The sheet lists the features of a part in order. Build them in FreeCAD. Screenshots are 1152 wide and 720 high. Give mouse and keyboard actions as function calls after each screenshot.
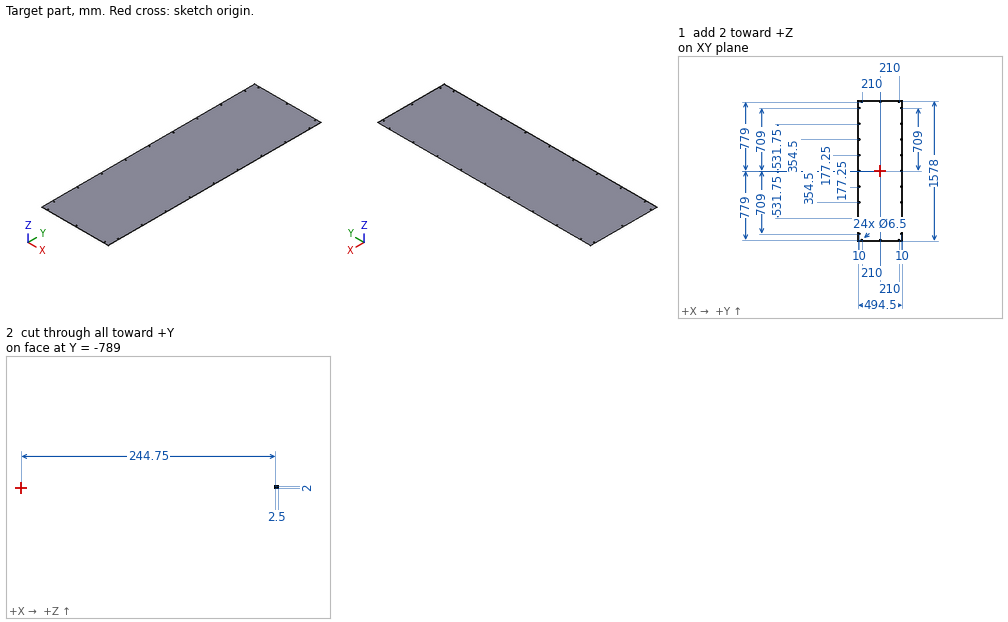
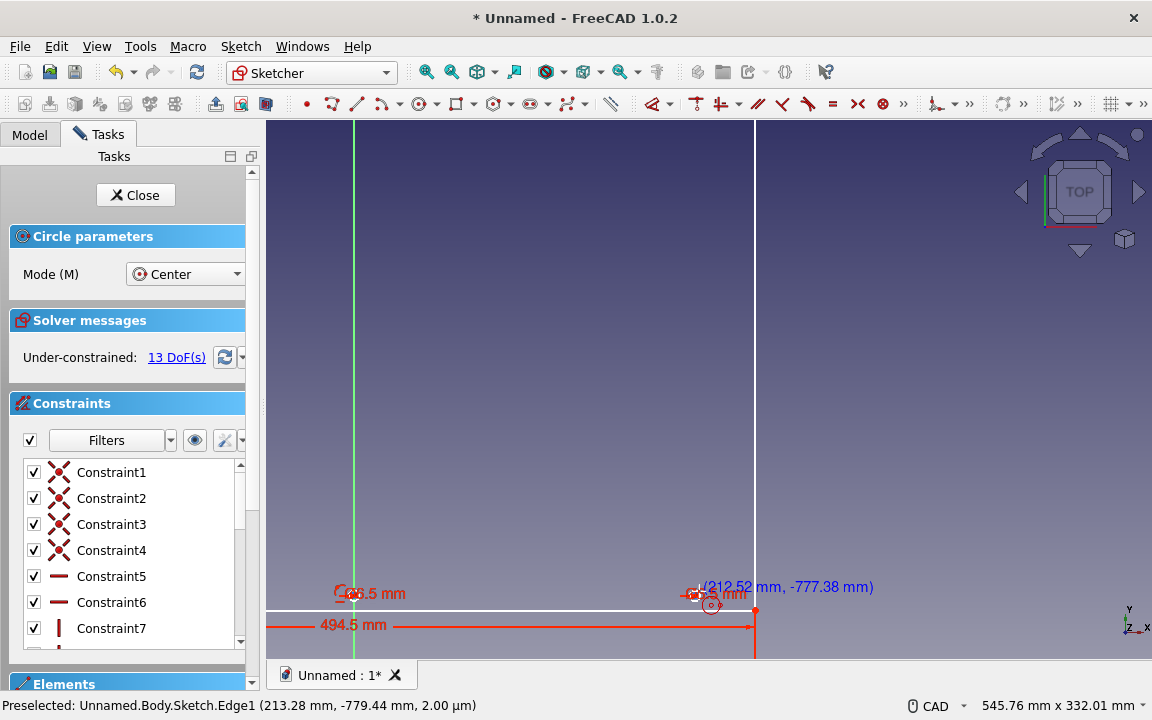
scroll(739, 481, up, 8)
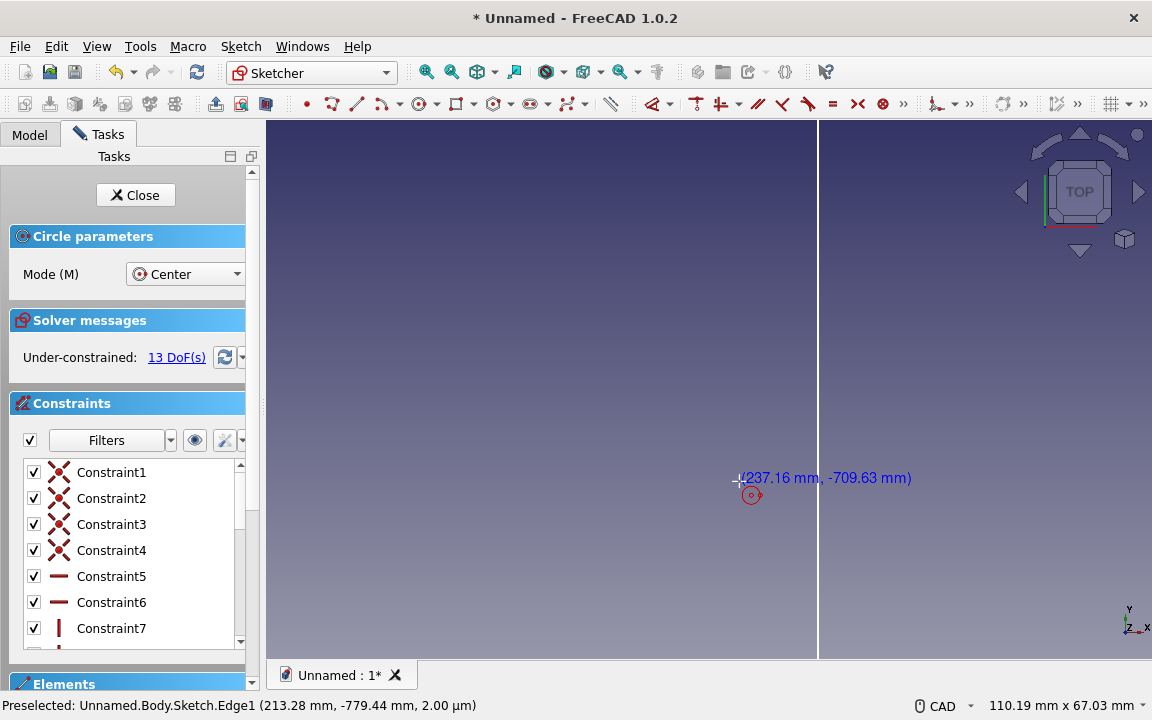
scroll(703, 583, down, 17)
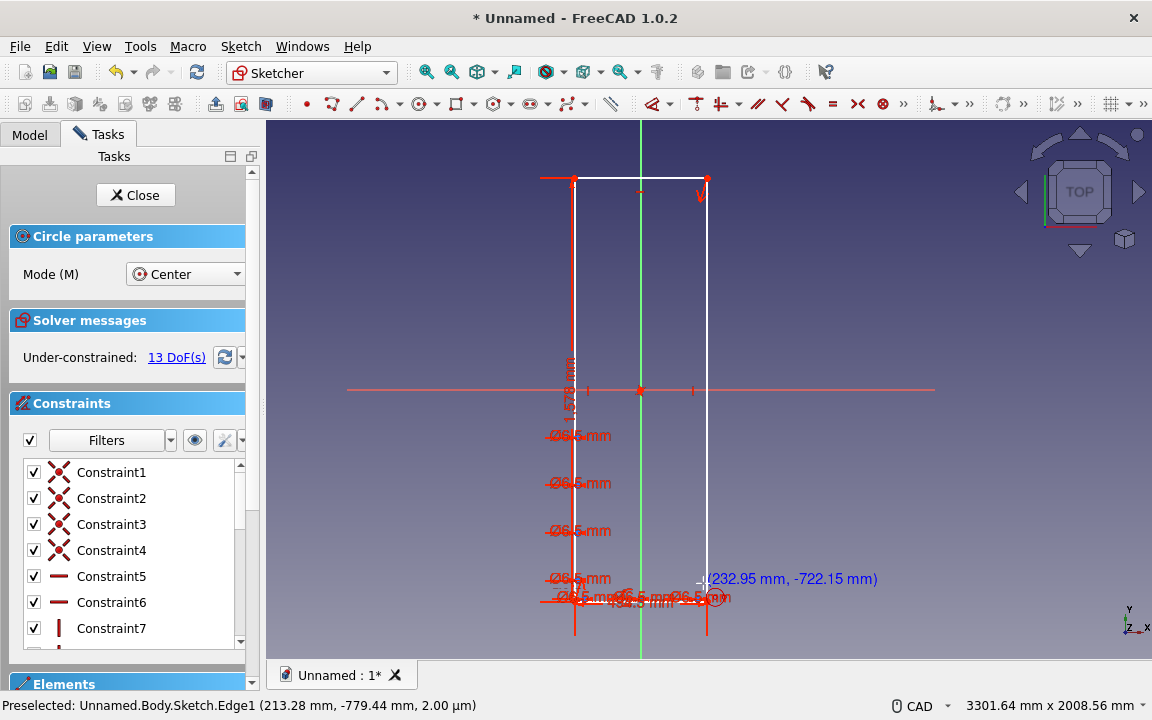
scroll(705, 580, up, 9)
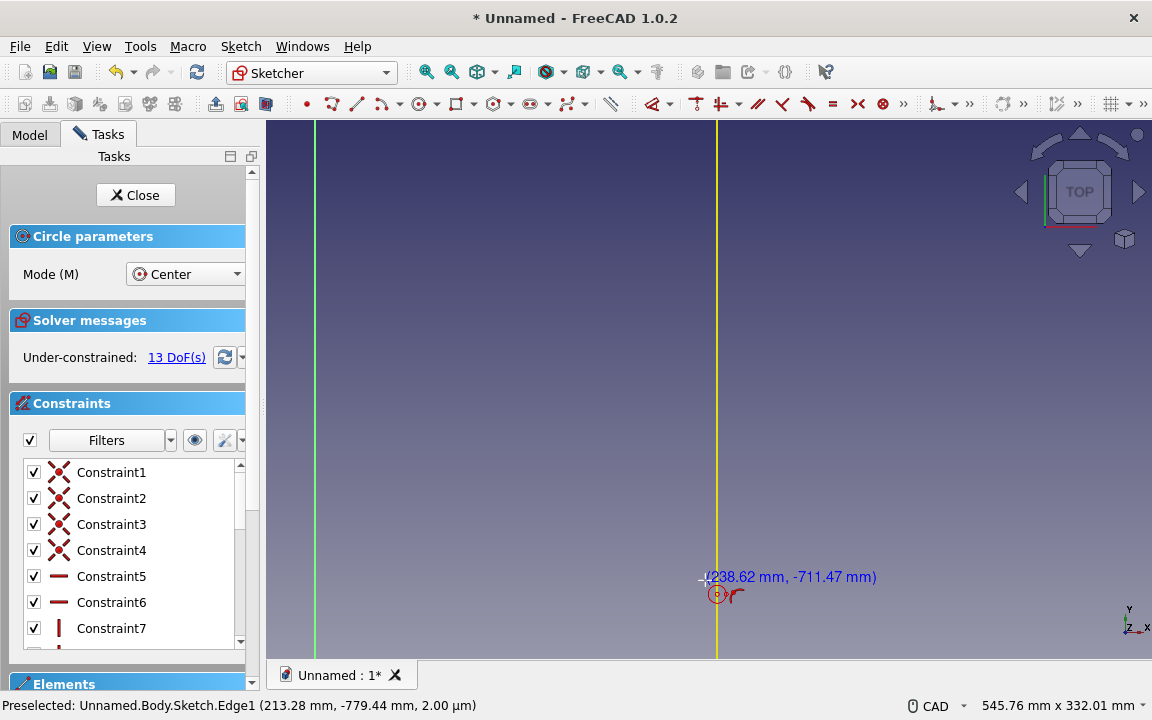
click(700, 578)
move(697, 574)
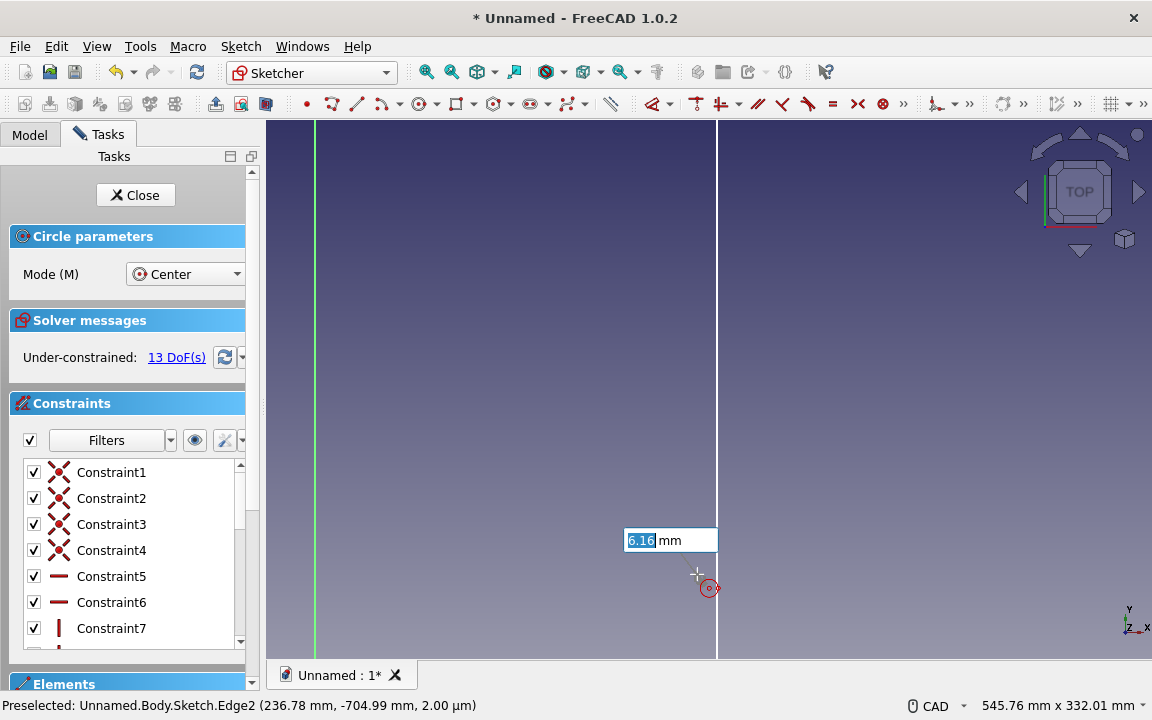
text(6.5)
key(Return)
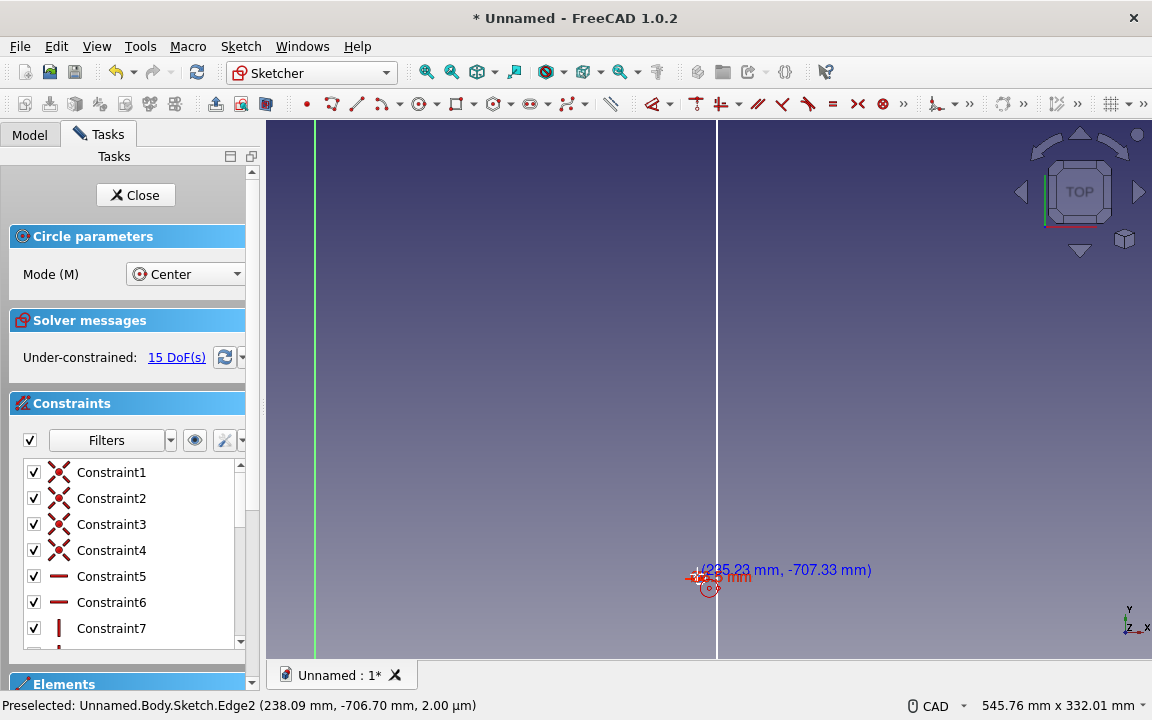
scroll(700, 290, up, 8)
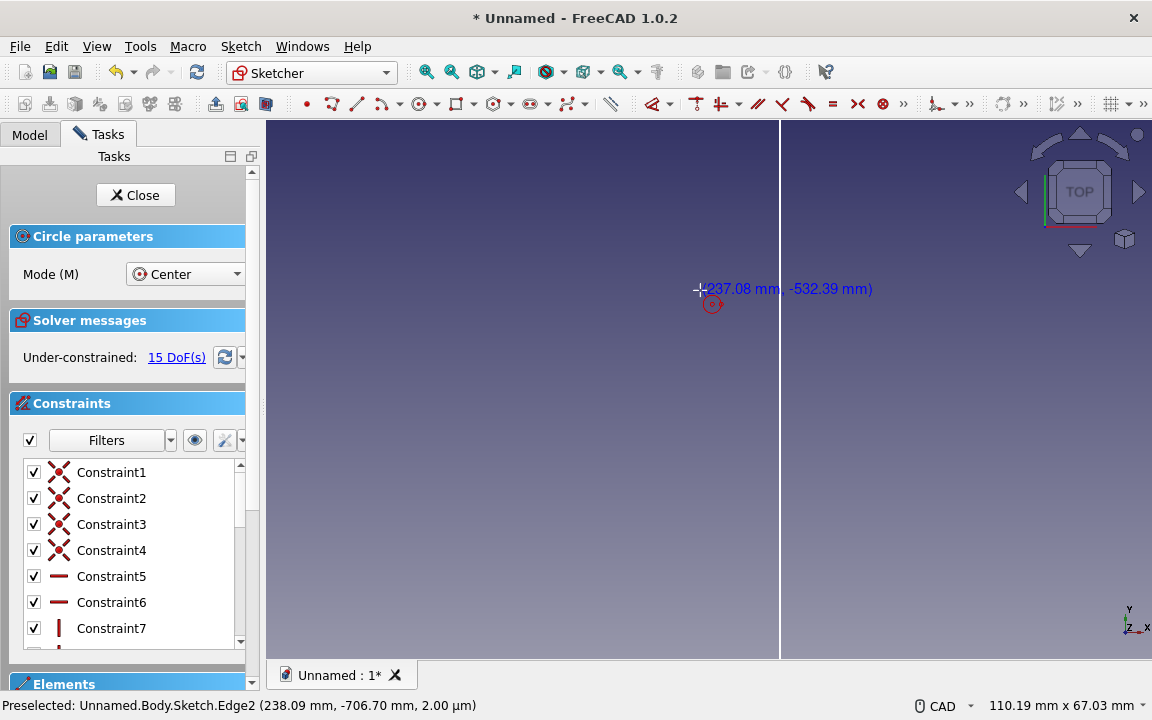
scroll(704, 541, down, 17)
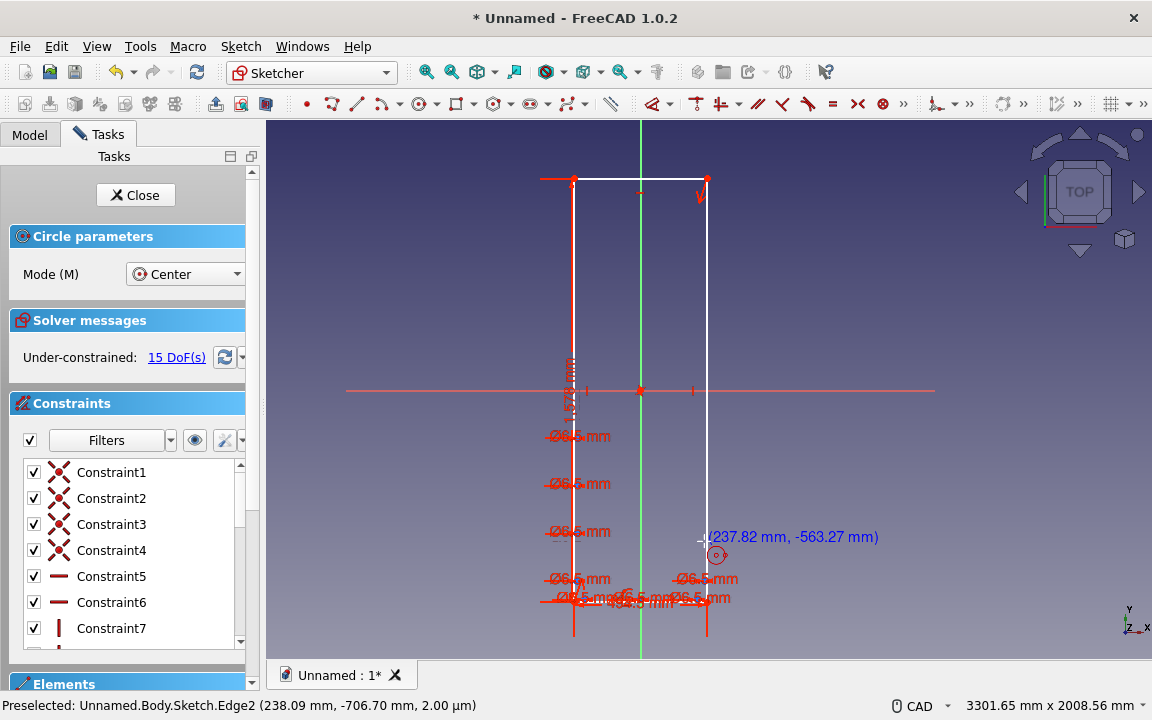
scroll(704, 533, up, 9)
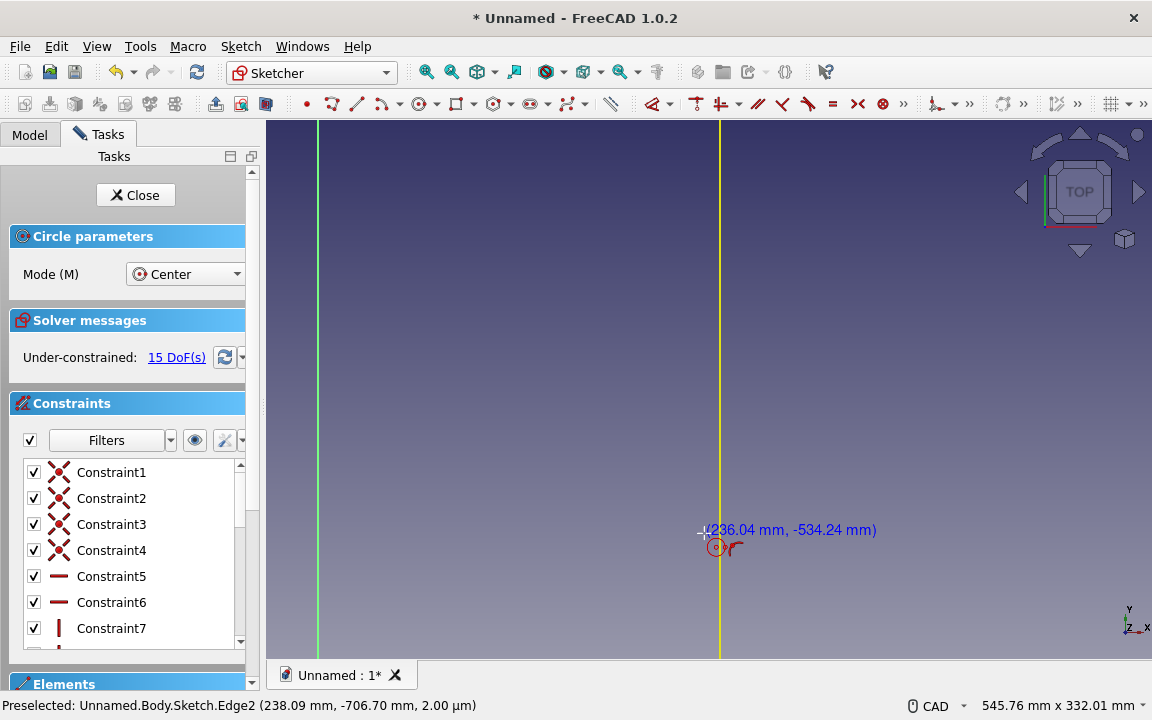
click(703, 531)
move(700, 527)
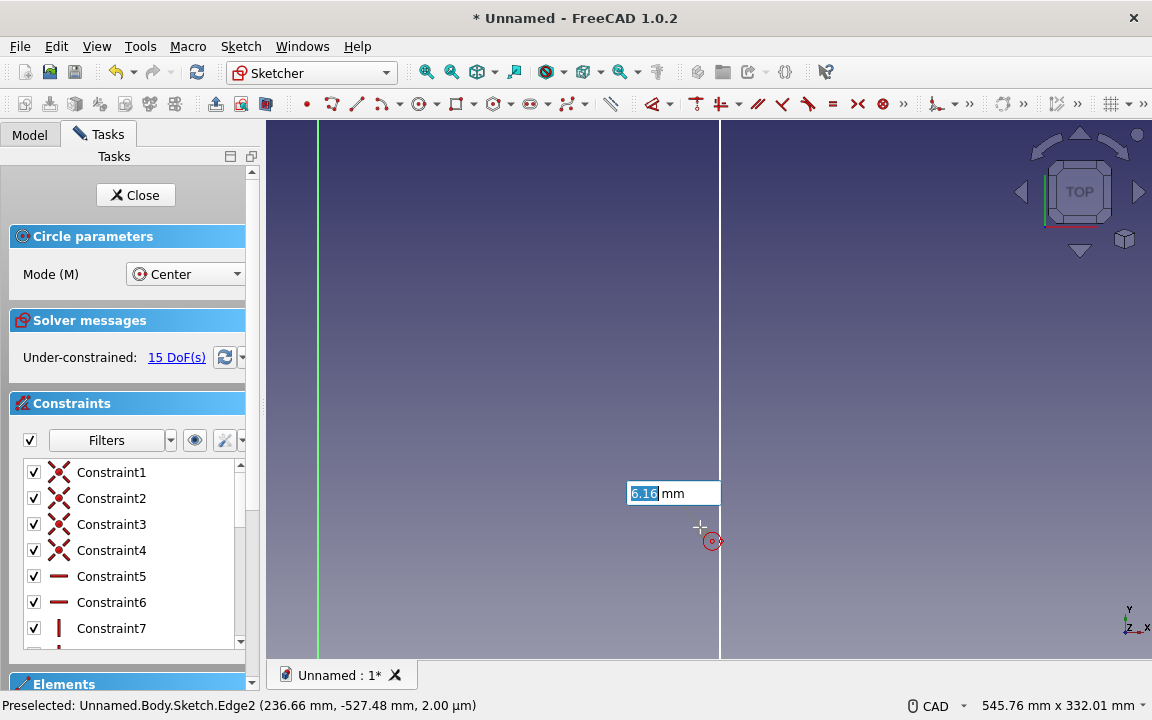
text(6.5)
key(Return)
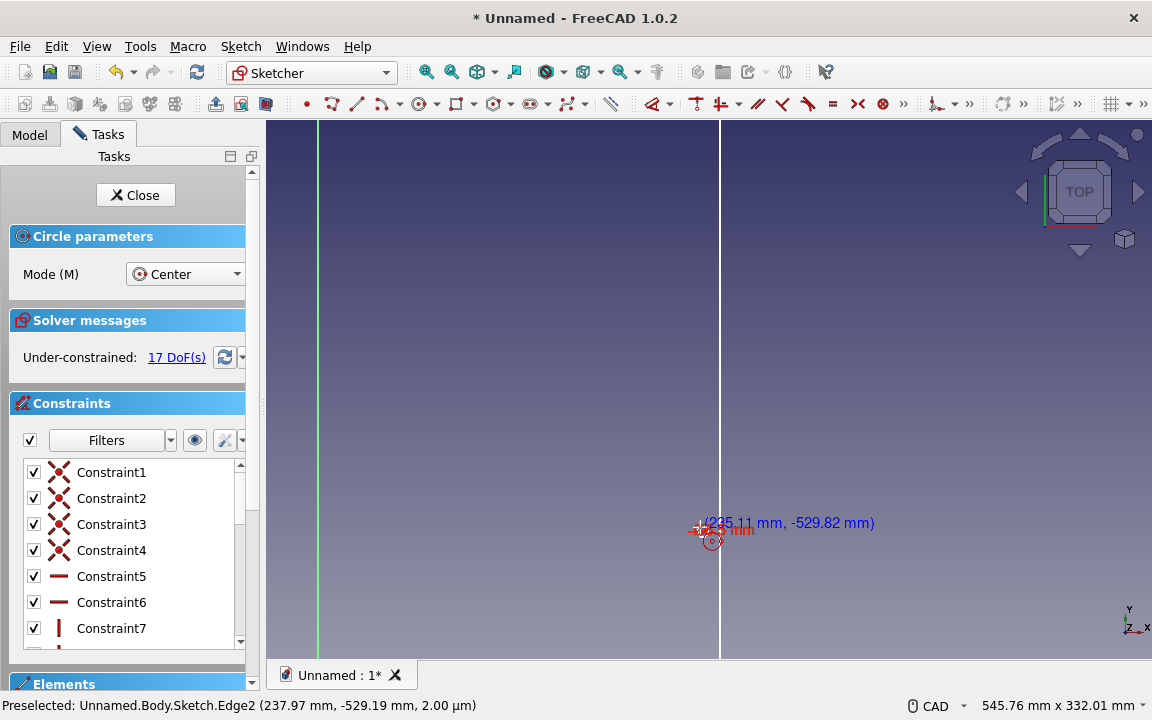
scroll(703, 243, up, 8)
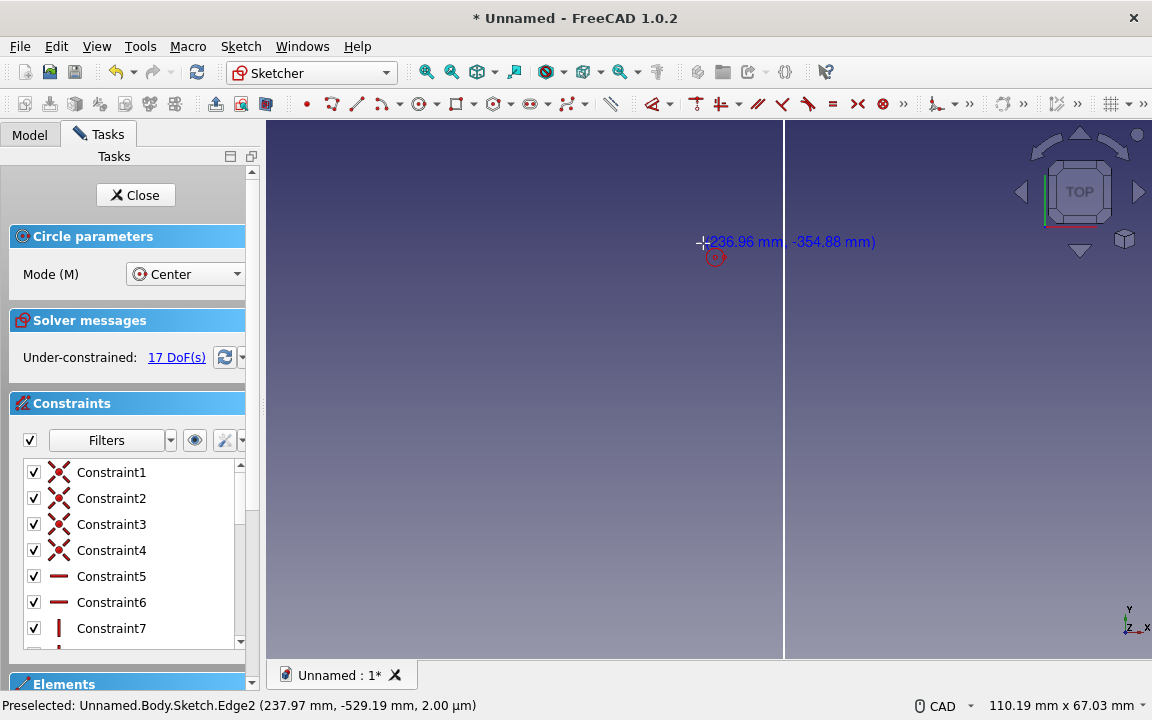
scroll(704, 493, down, 17)